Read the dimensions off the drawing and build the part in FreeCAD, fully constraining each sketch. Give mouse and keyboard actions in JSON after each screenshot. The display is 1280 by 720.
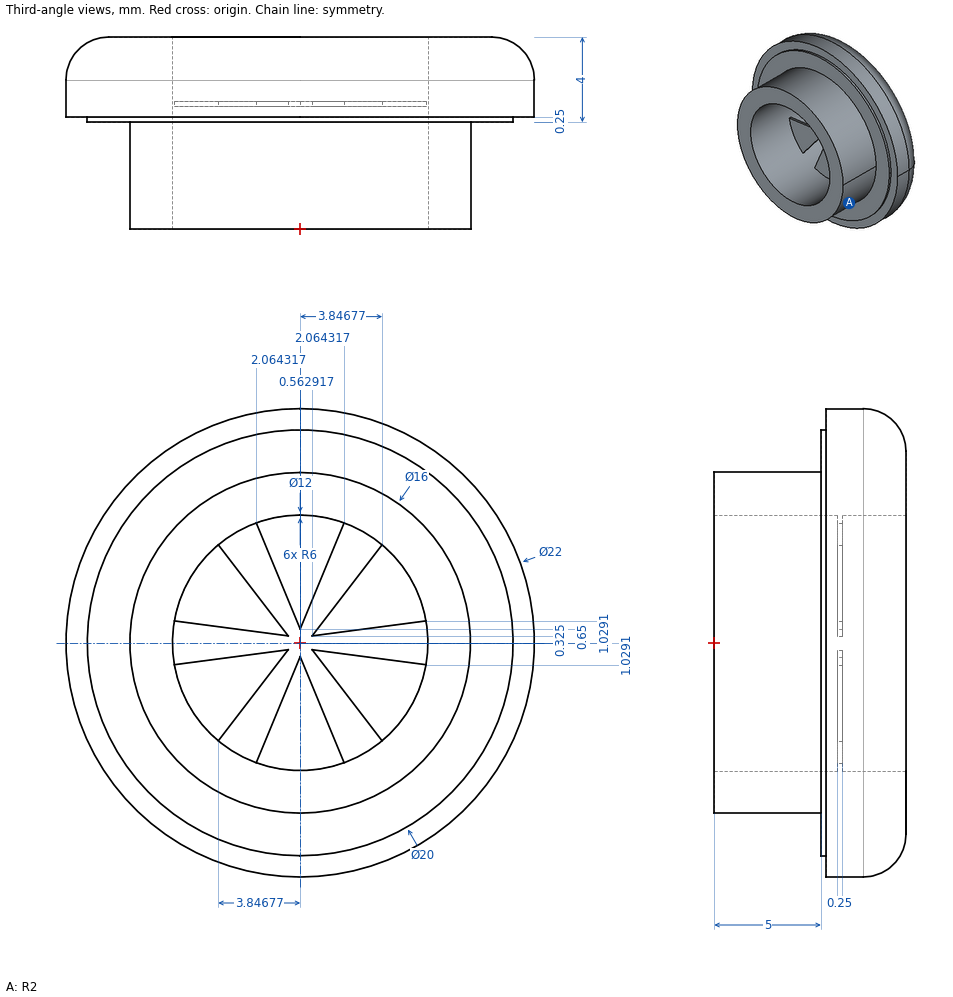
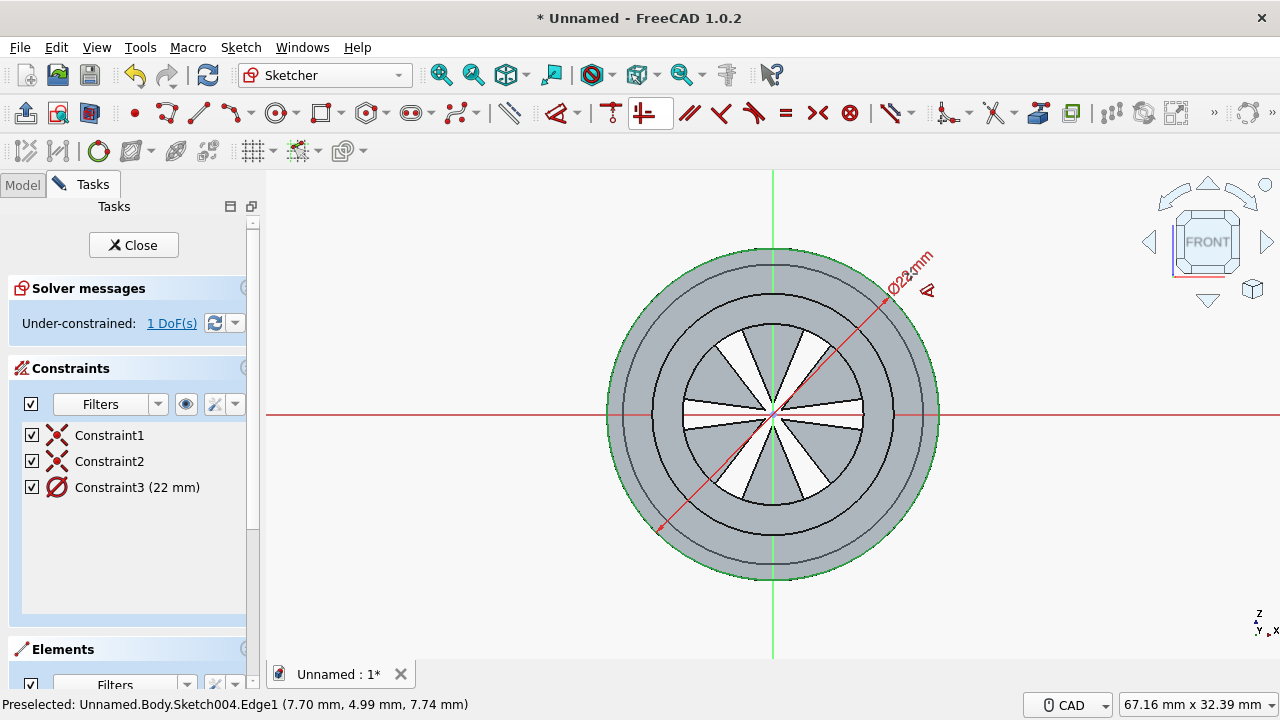
{"action": "left_click", "coordinate": [879, 308]}
{"action": "left_click", "coordinate": [948, 363]}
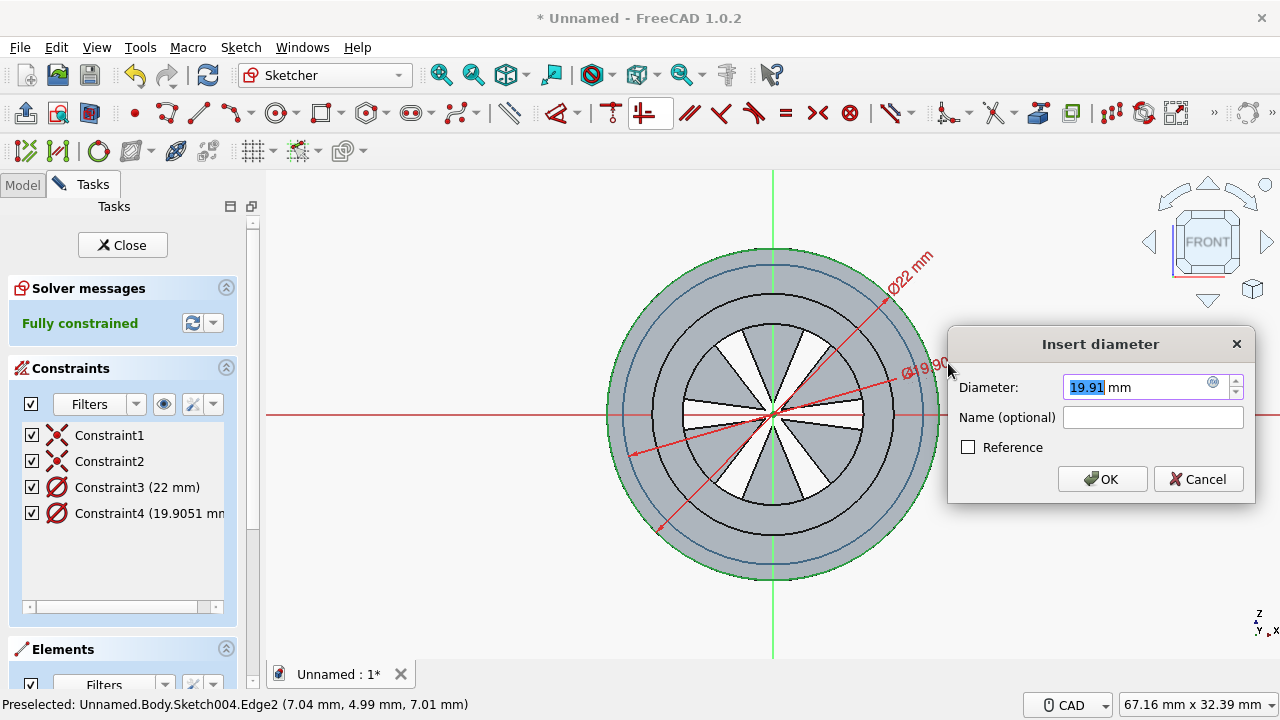
{"action": "type", "text": "20"}
{"action": "key", "text": "Return"}
{"action": "key", "text": "Escape"}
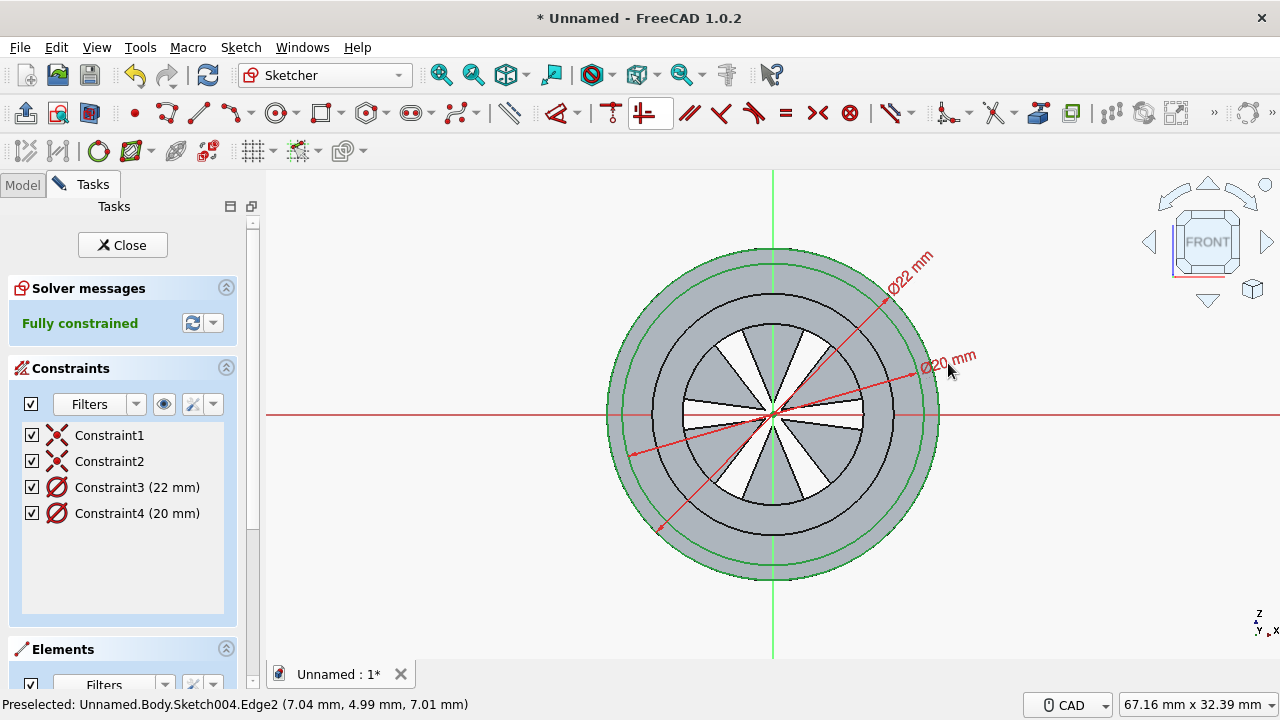
{"action": "left_click", "coordinate": [123, 245]}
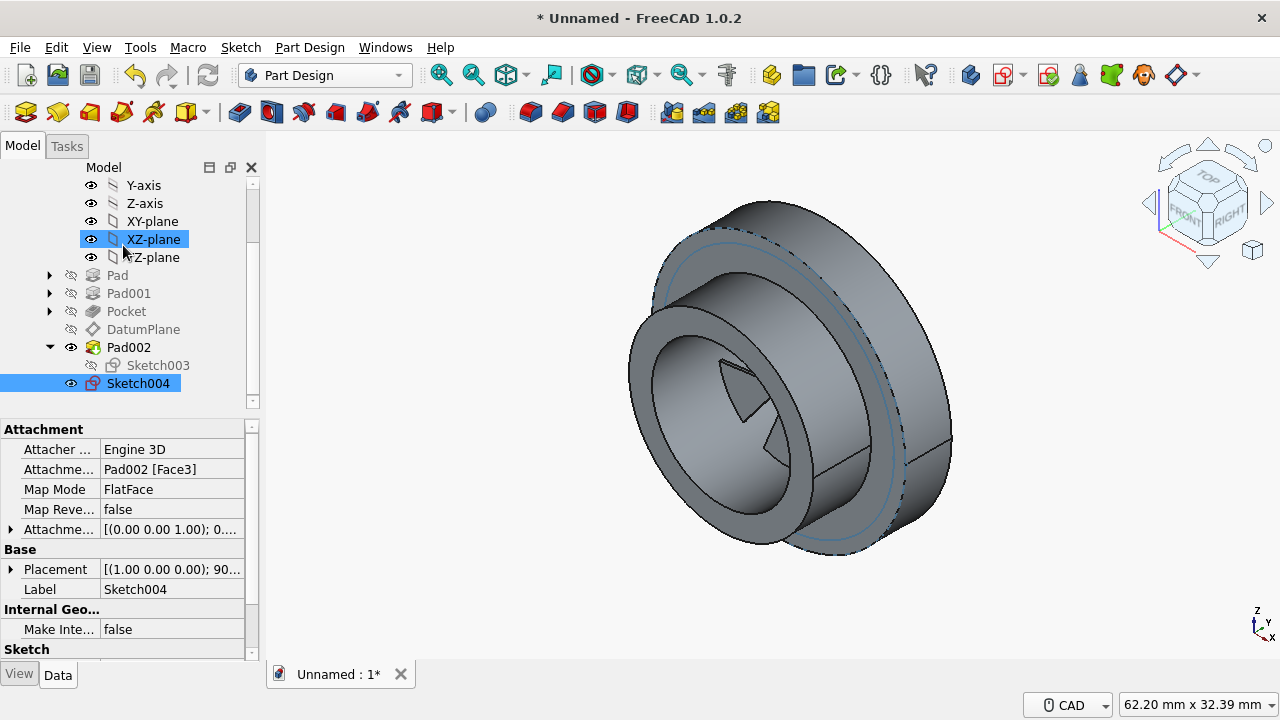
{"action": "left_click", "coordinate": [240, 112]}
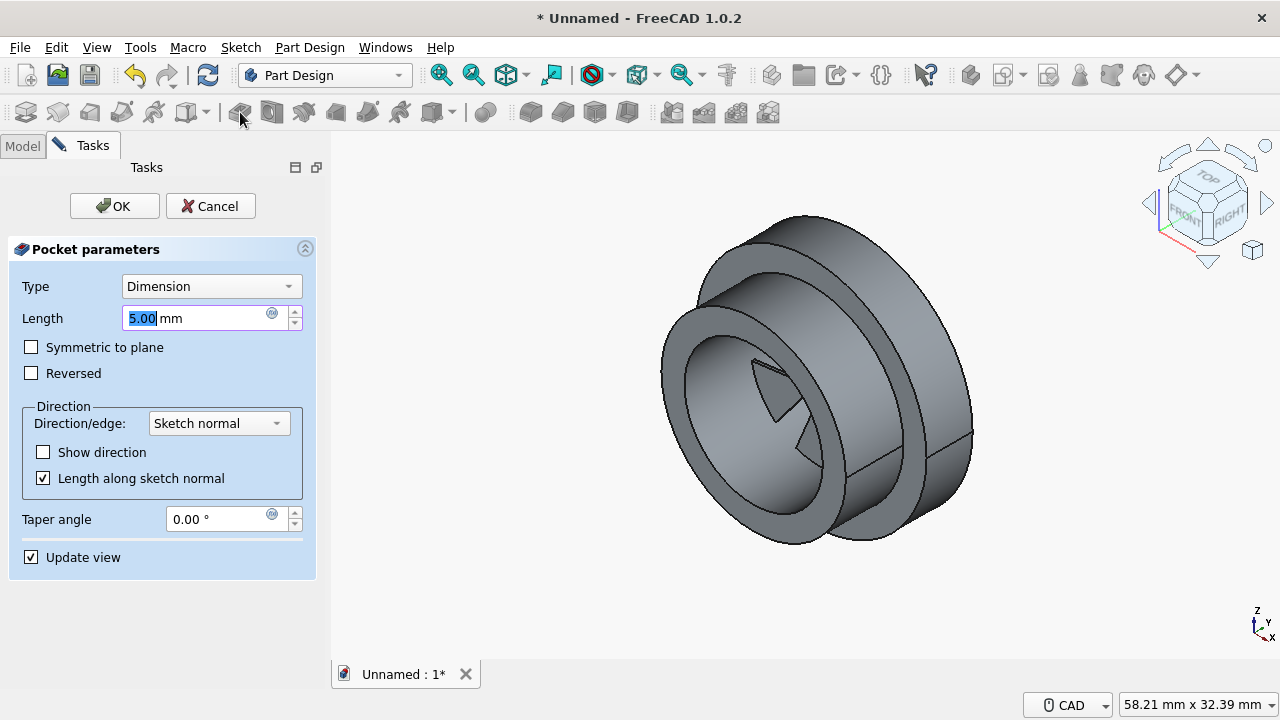
{"action": "type", "text": "0.25"}
{"action": "key", "text": "Tab"}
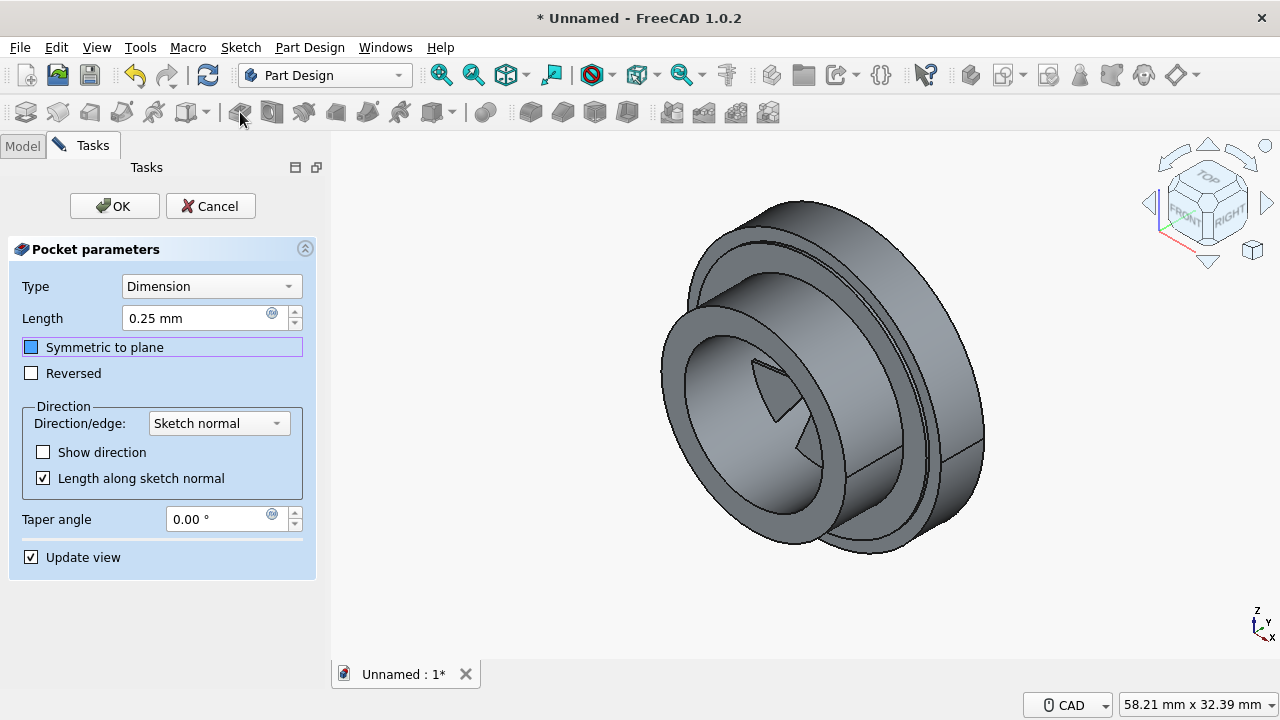
{"action": "left_click", "coordinate": [115, 206]}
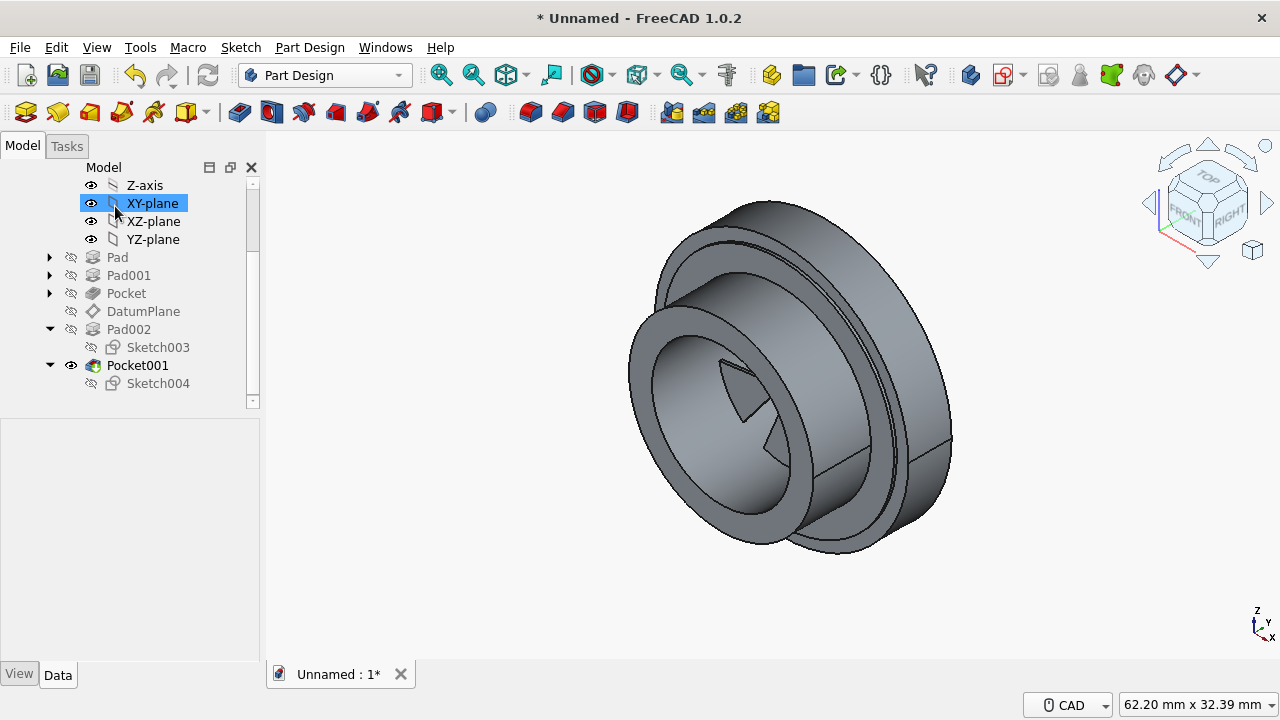
{"action": "left_click", "coordinate": [864, 247]}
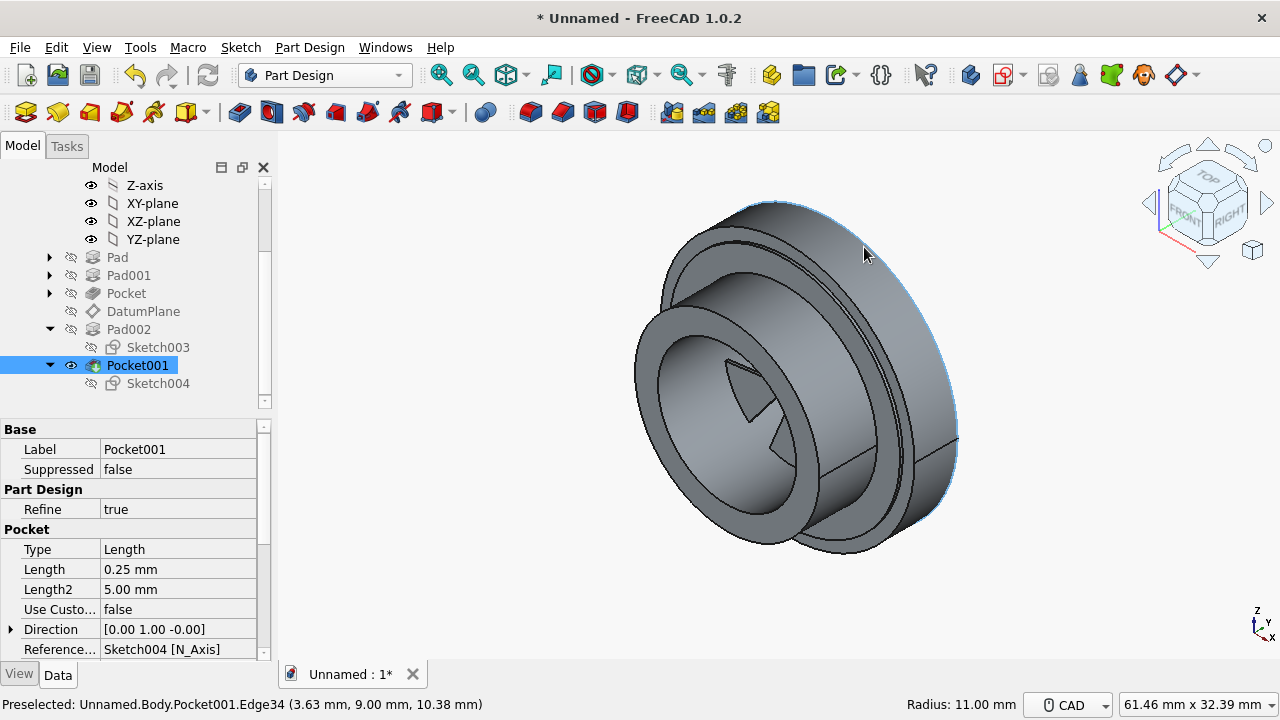
{"action": "left_click", "coordinate": [532, 112]}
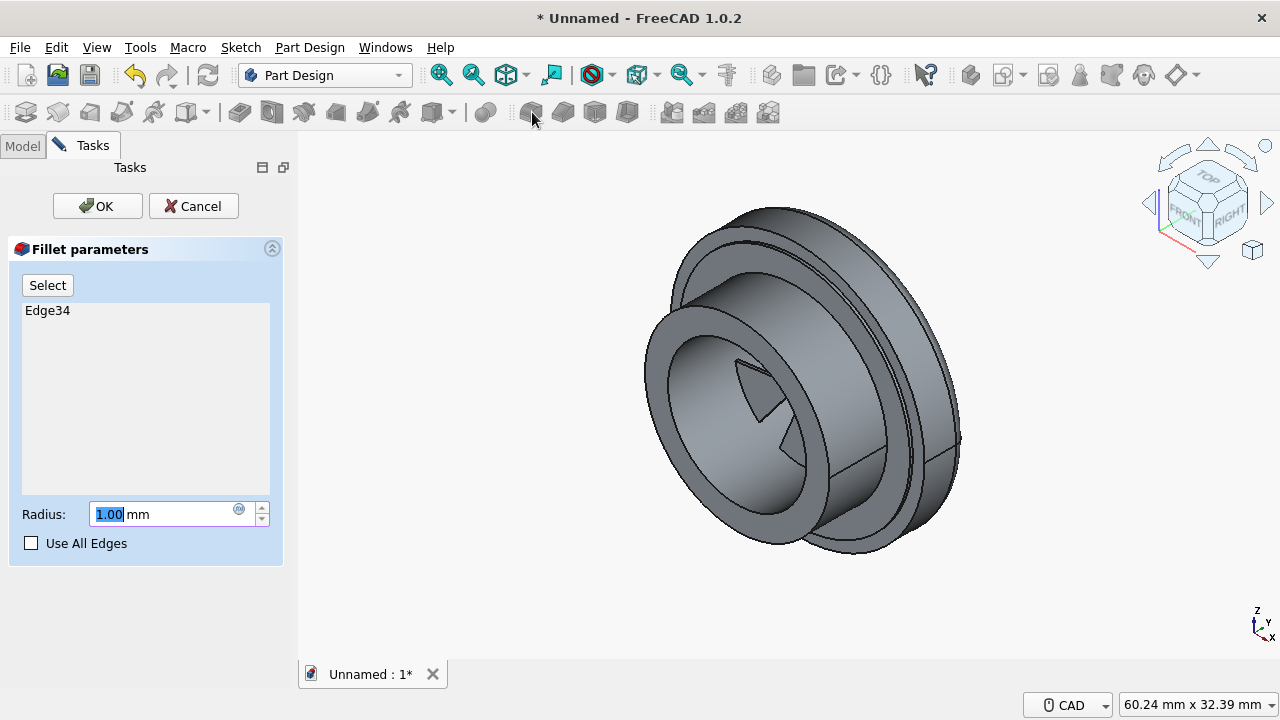
{"action": "type", "text": "2"}
{"action": "key", "text": "Tab"}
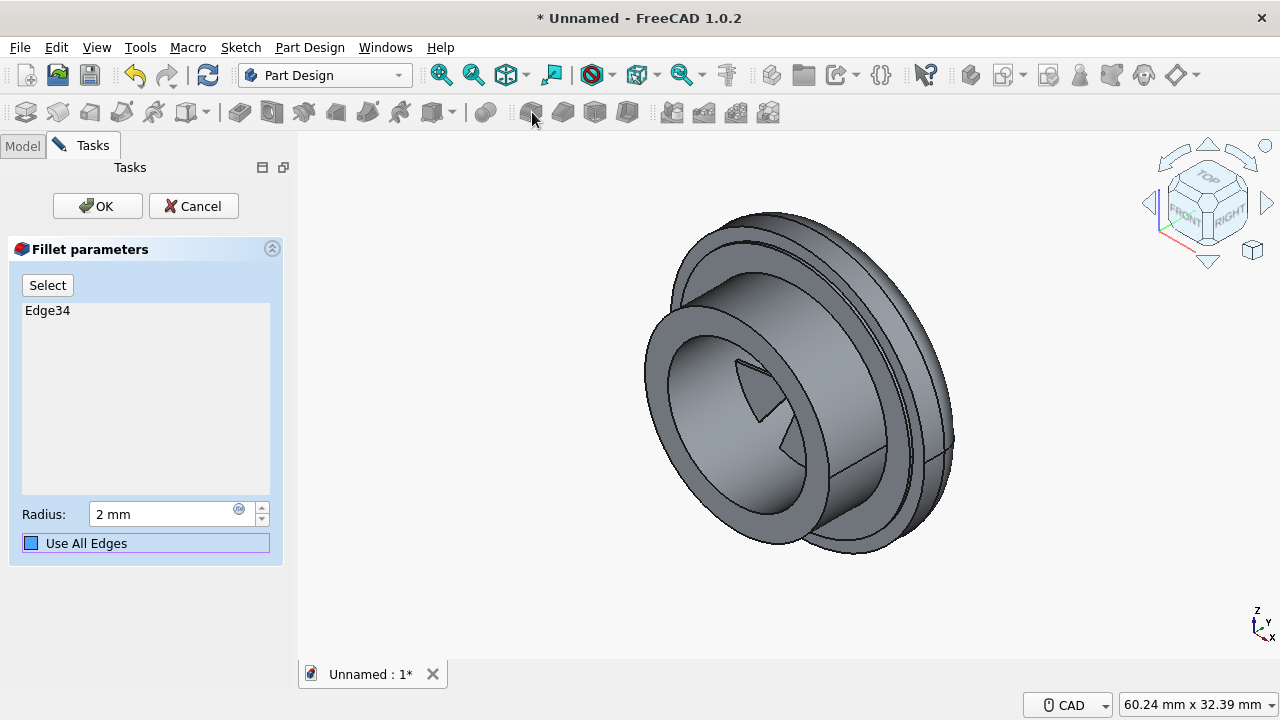
{"action": "left_click", "coordinate": [98, 206]}